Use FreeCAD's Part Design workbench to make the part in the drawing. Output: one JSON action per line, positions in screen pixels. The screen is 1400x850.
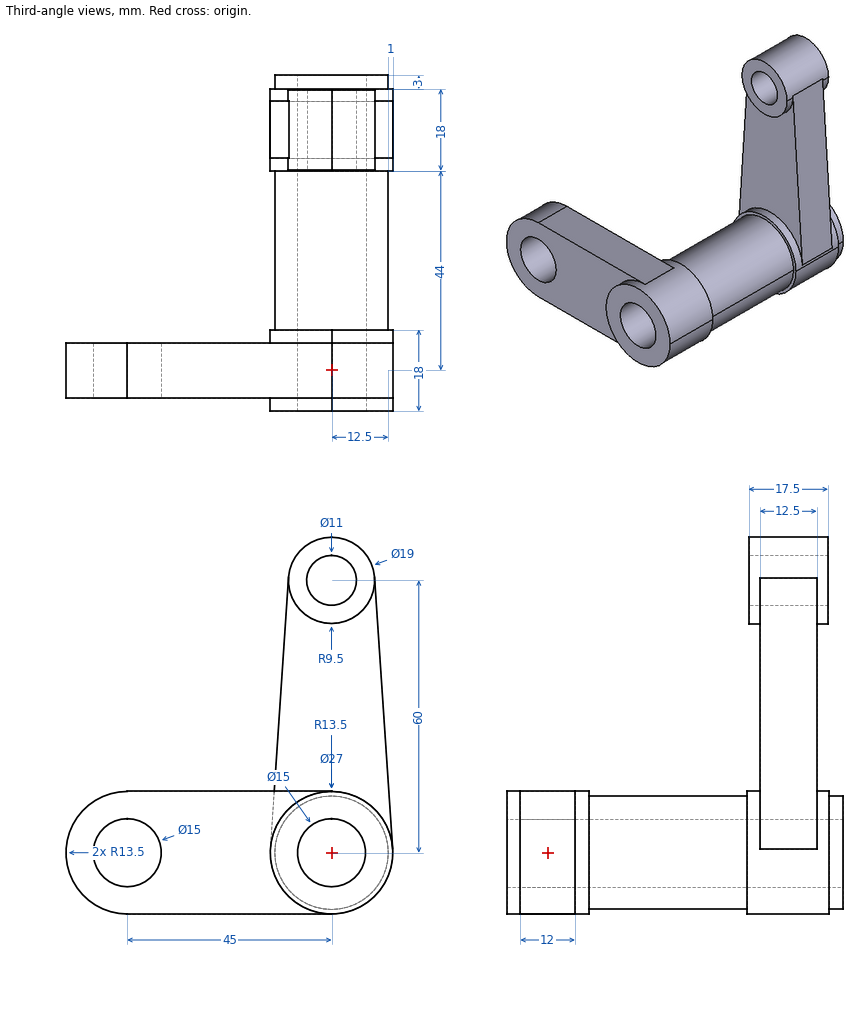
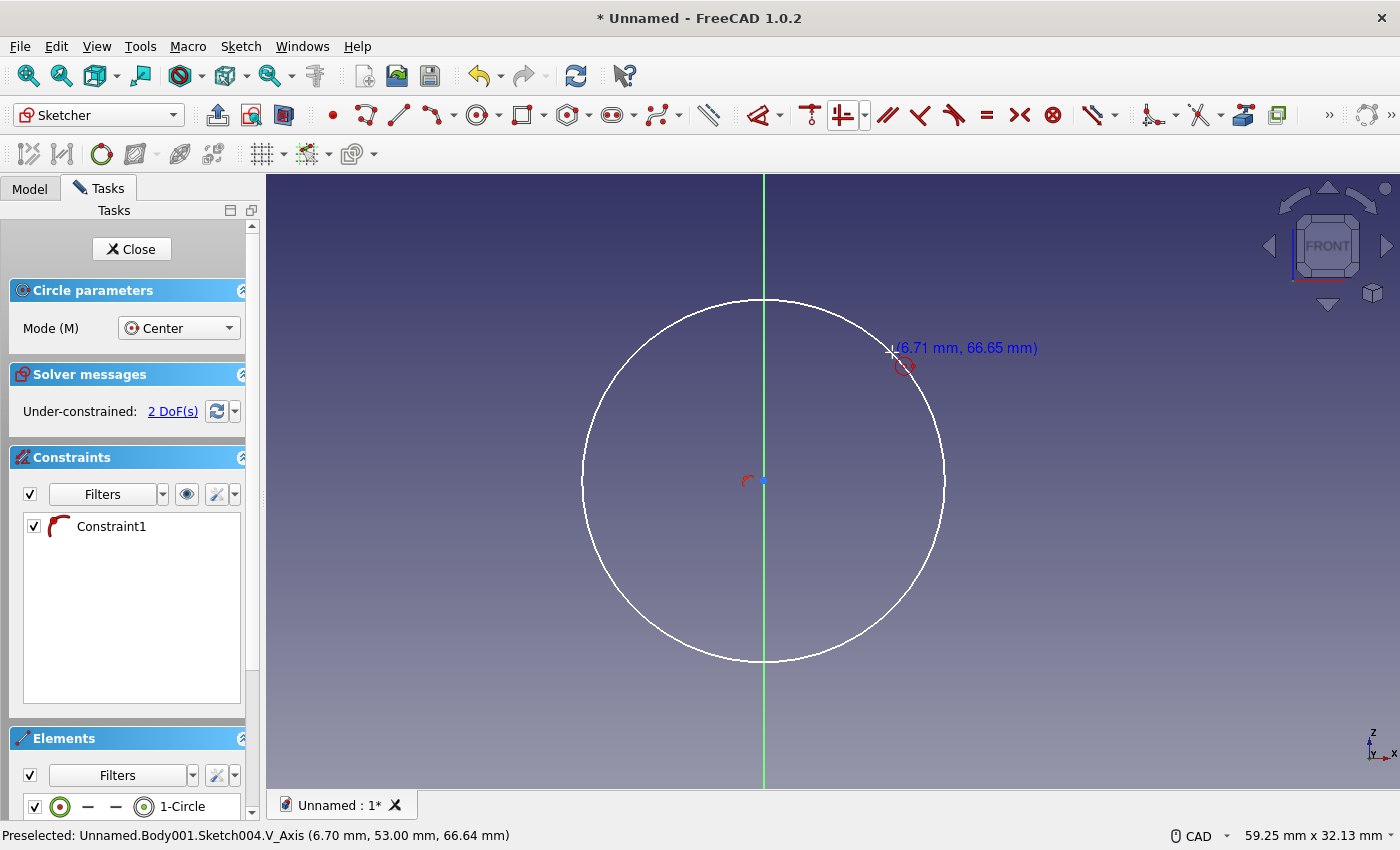
{"action": "left_click", "coordinate": [764, 481]}
{"action": "left_click", "coordinate": [838, 406]}
{"action": "key", "text": "Escape"}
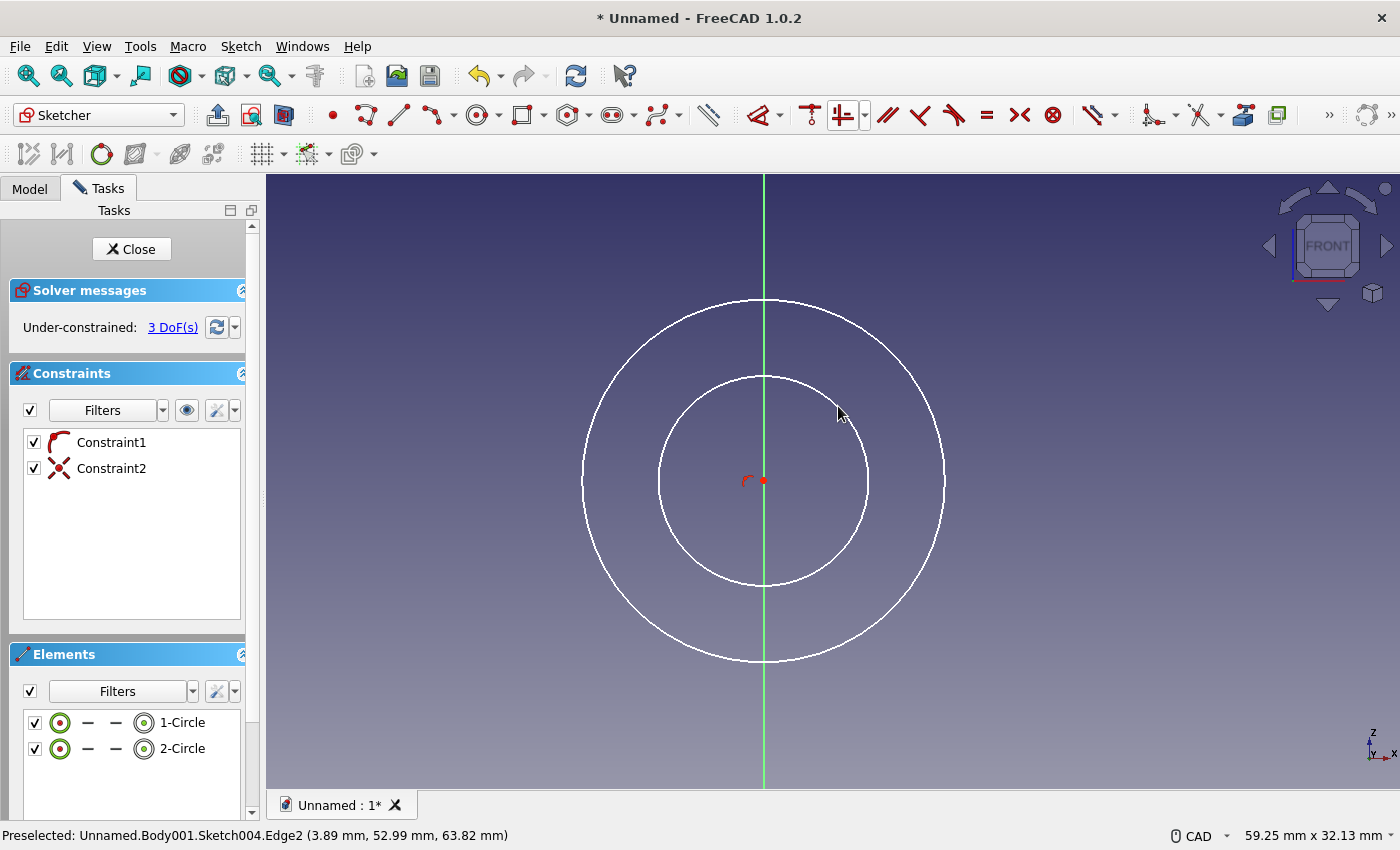
{"action": "left_click", "coordinate": [758, 116]}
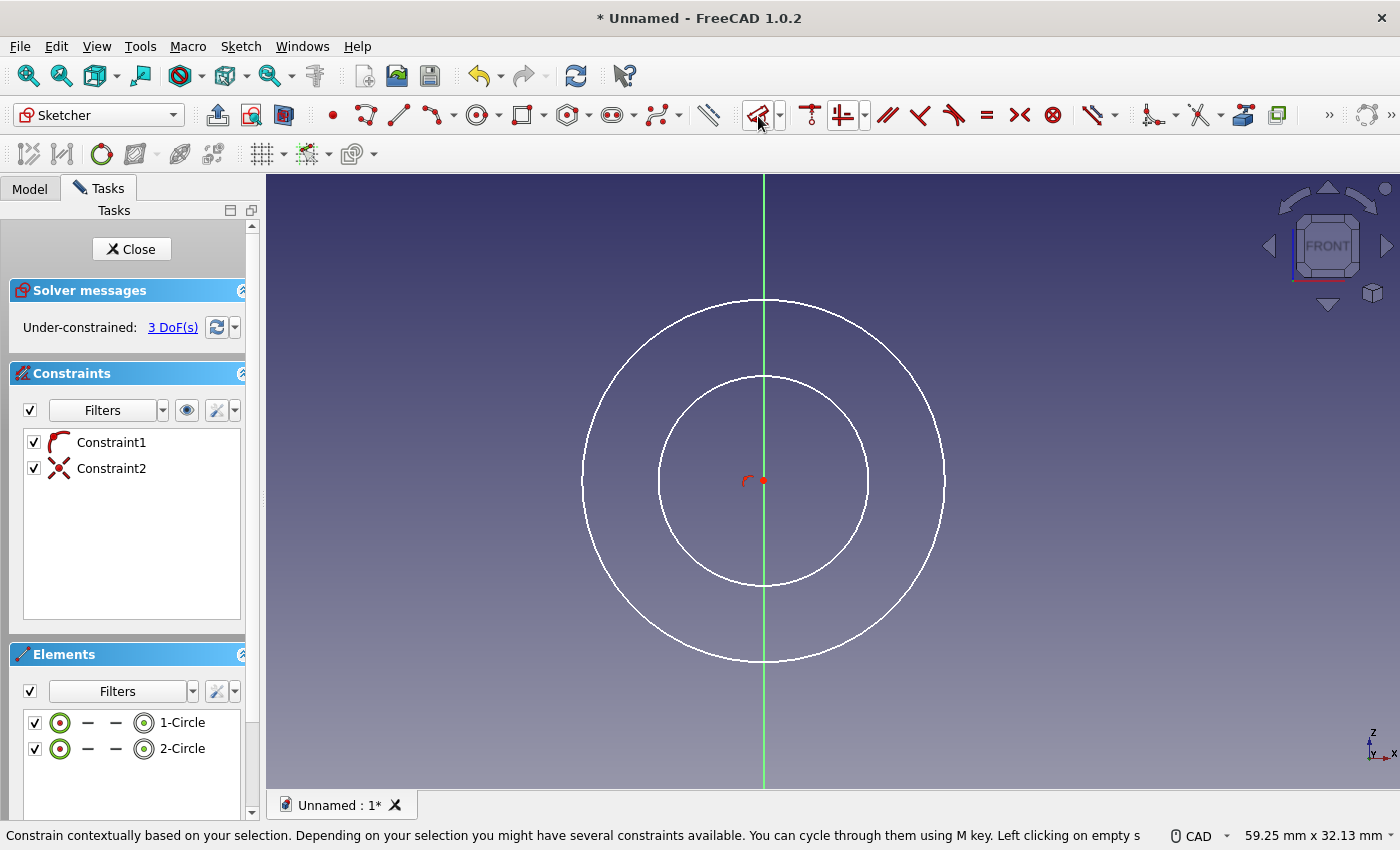
{"action": "left_click", "coordinate": [891, 352]}
{"action": "left_click", "coordinate": [913, 329]}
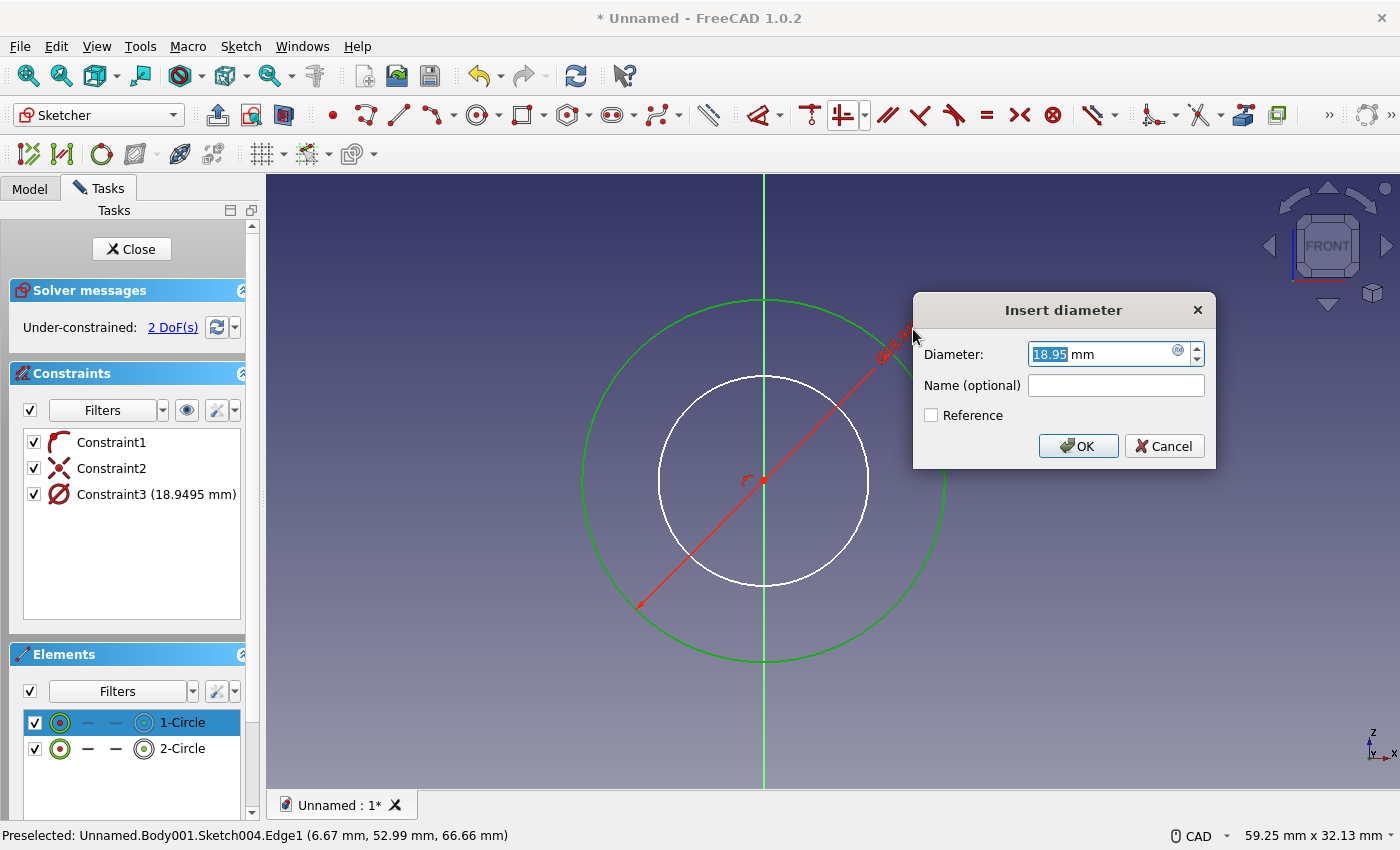
{"action": "type", "text": "19"}
{"action": "key", "text": "Return"}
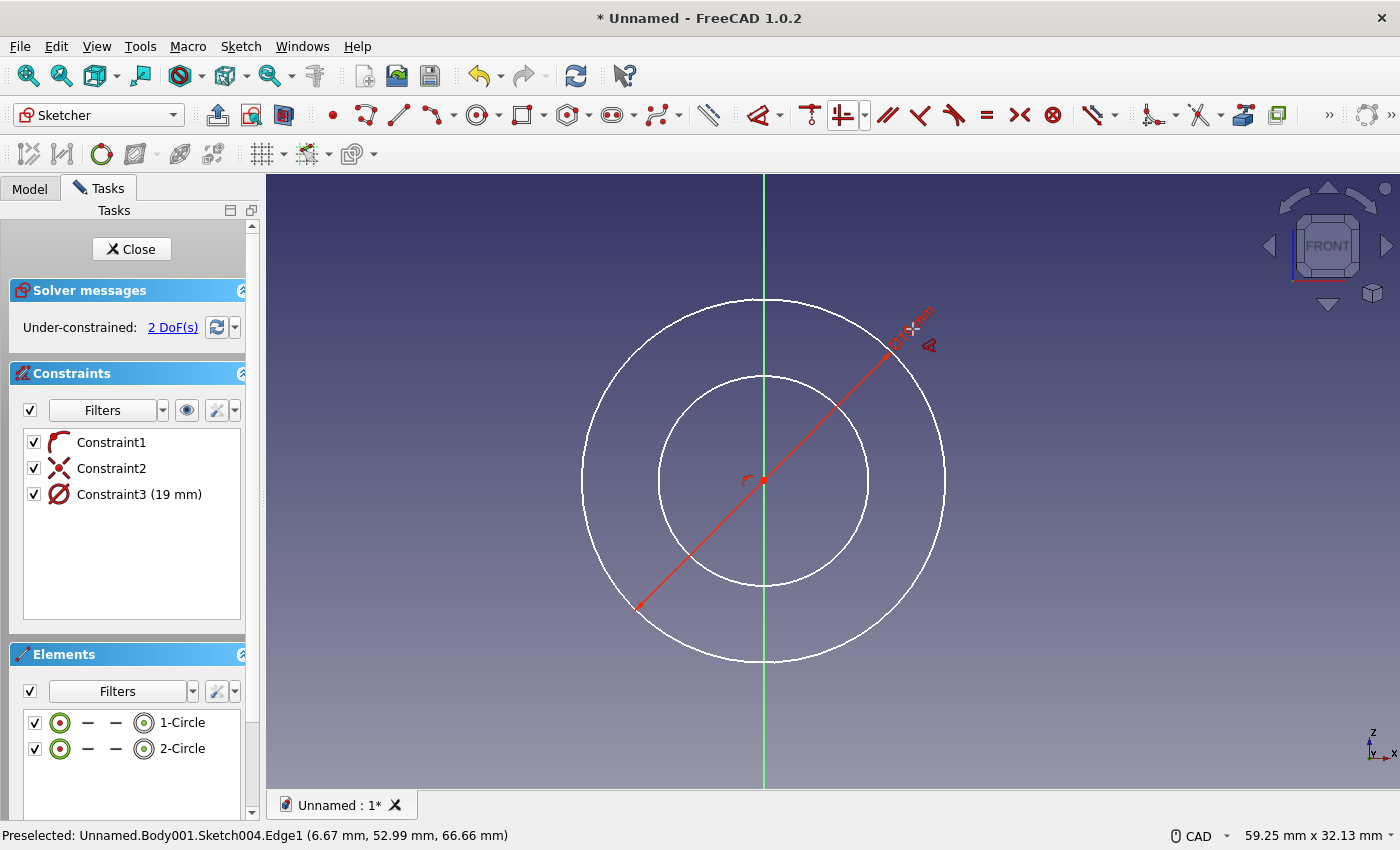
{"action": "left_click", "coordinate": [838, 407]}
{"action": "left_click", "coordinate": [861, 384]}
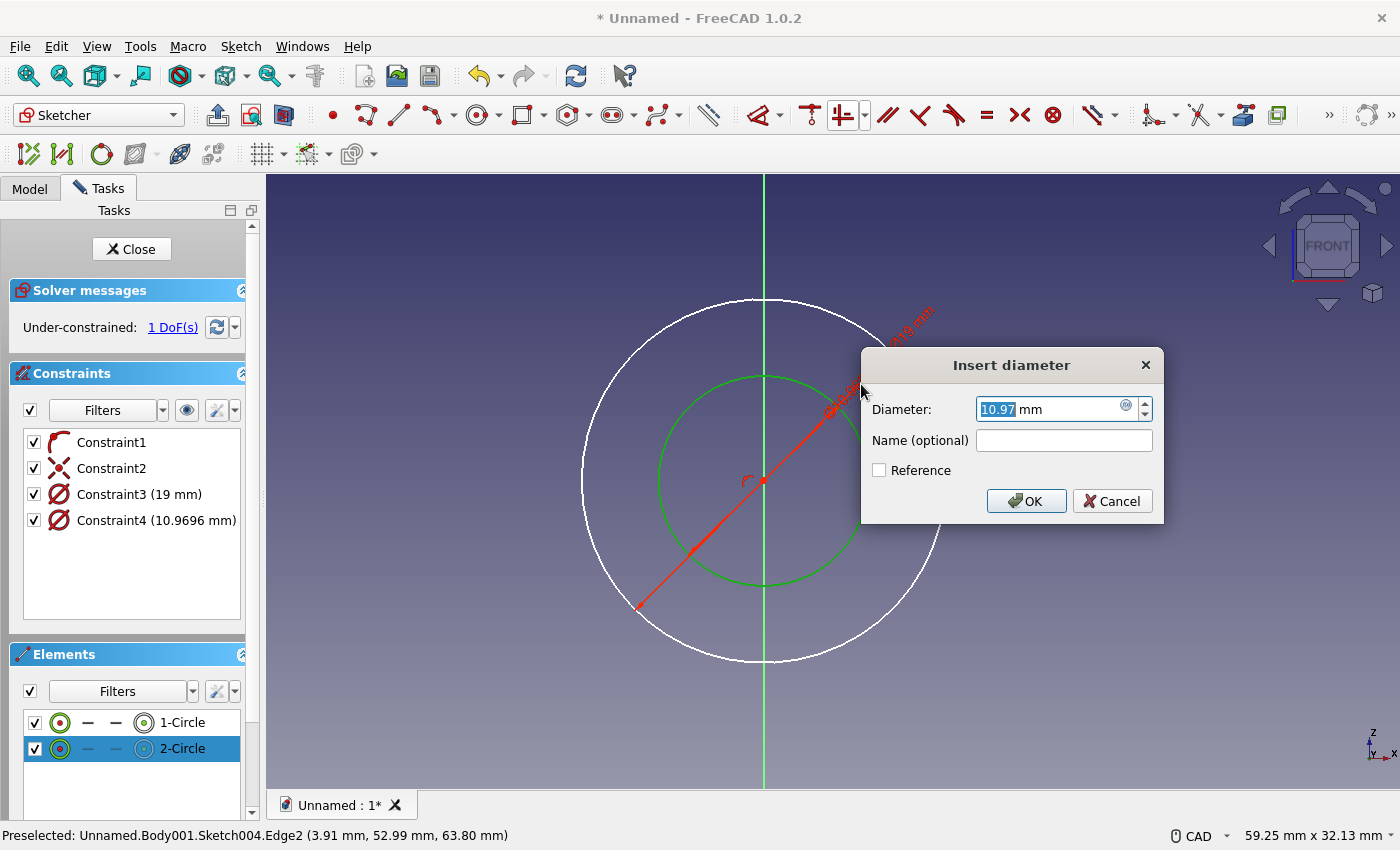
{"action": "type", "text": "11"}
{"action": "key", "text": "Return"}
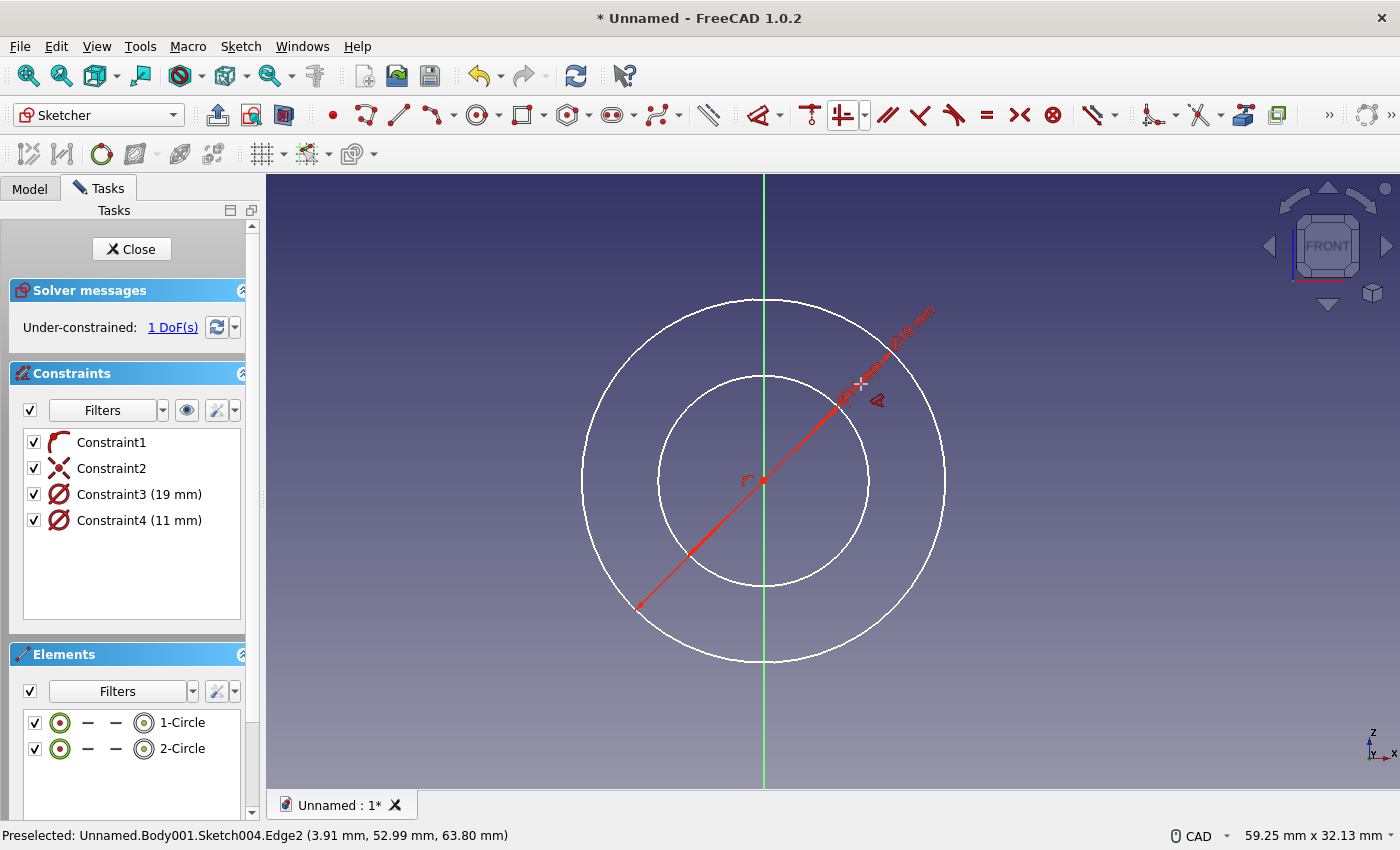
{"action": "left_click", "coordinate": [764, 481]}
{"action": "left_click", "coordinate": [798, 621]}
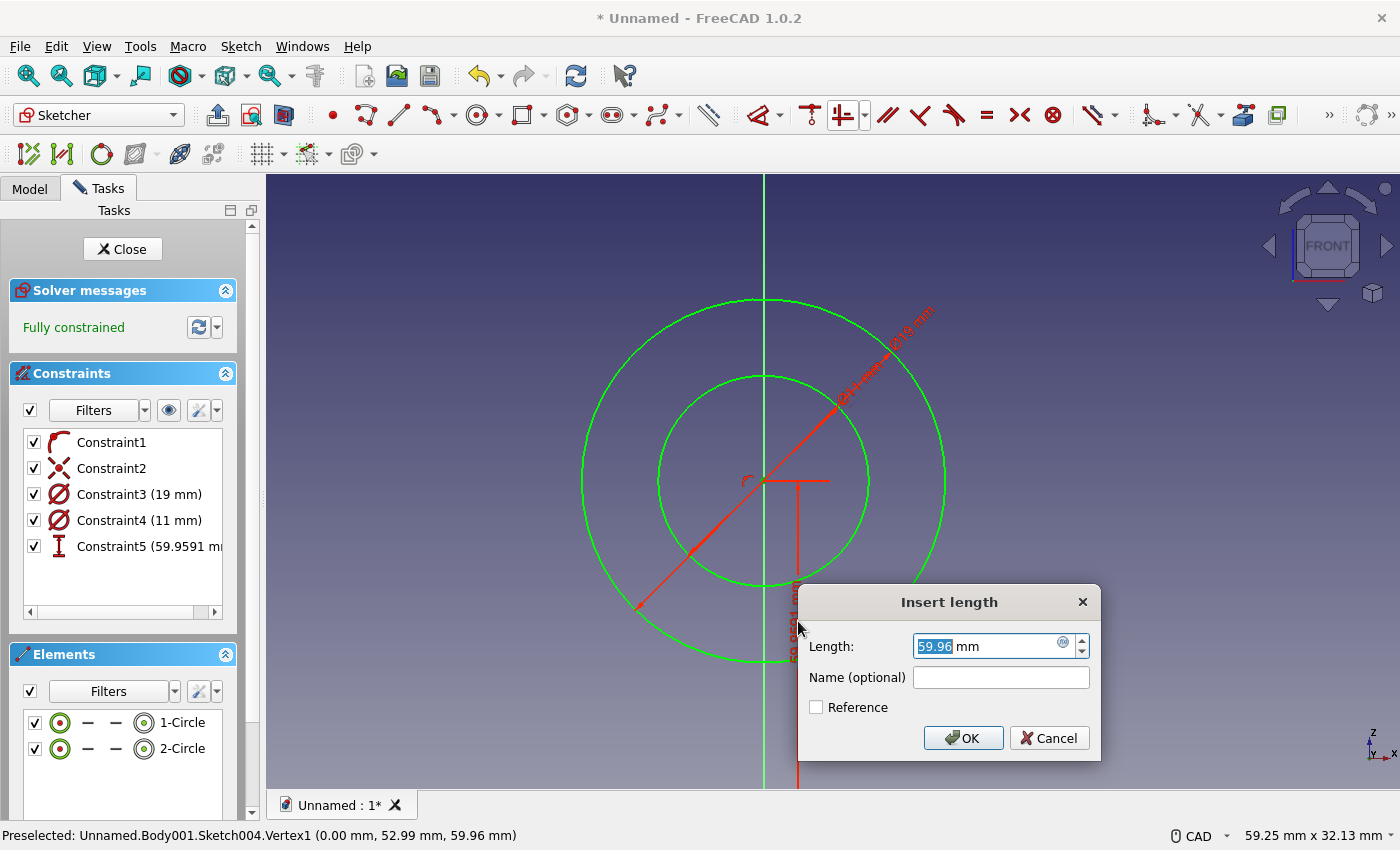
{"action": "type", "text": "60"}
{"action": "key", "text": "Return"}
{"action": "key", "text": "Escape"}